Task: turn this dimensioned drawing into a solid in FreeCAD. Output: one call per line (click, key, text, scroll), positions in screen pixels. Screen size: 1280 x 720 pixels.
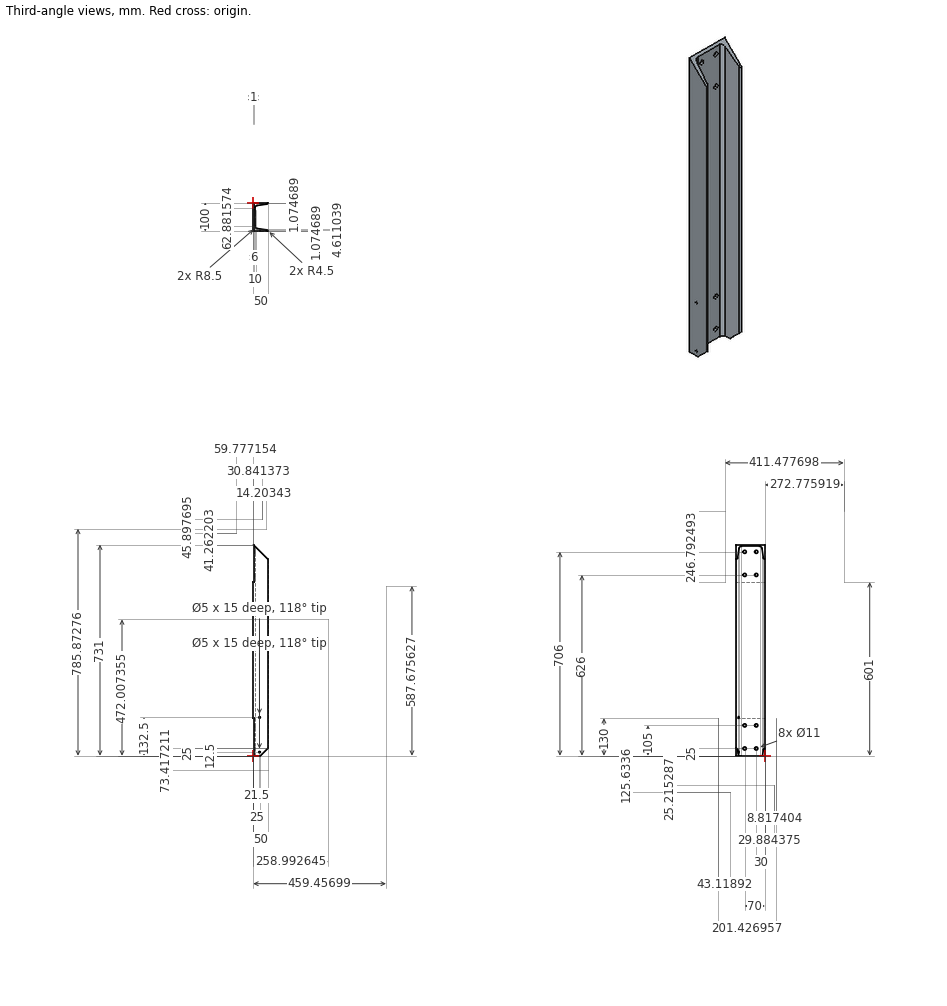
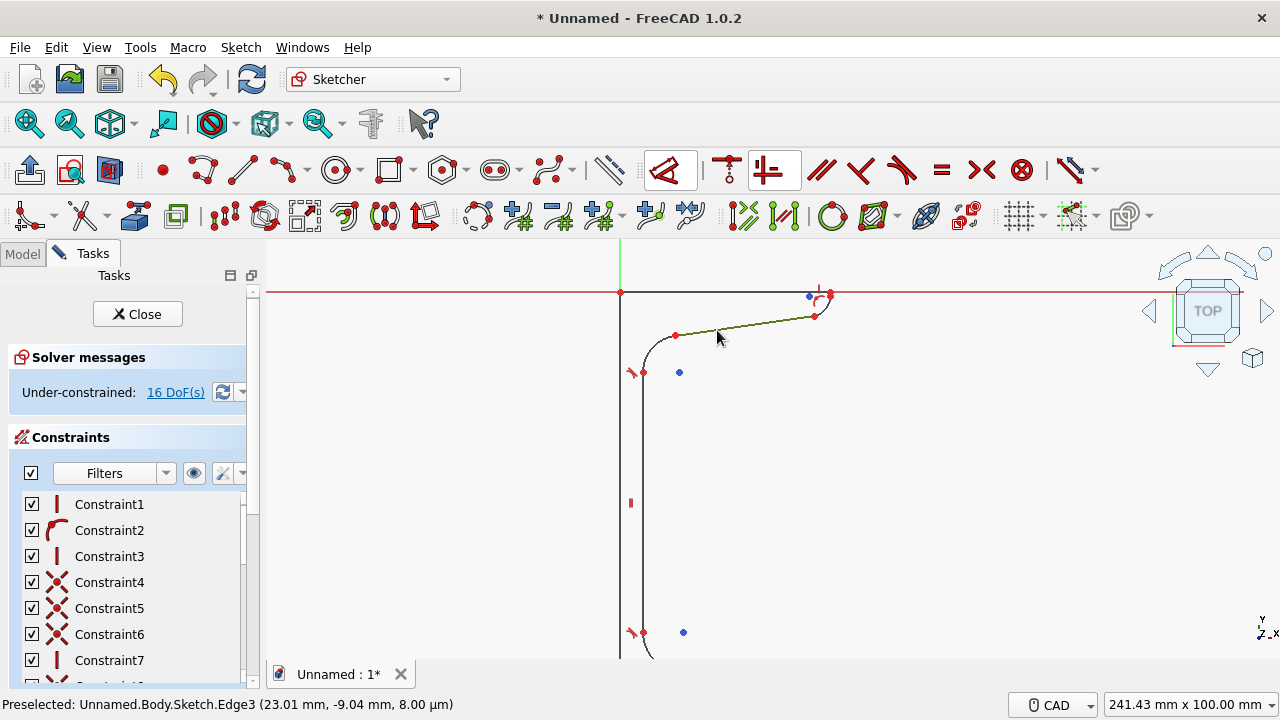
click(660, 341)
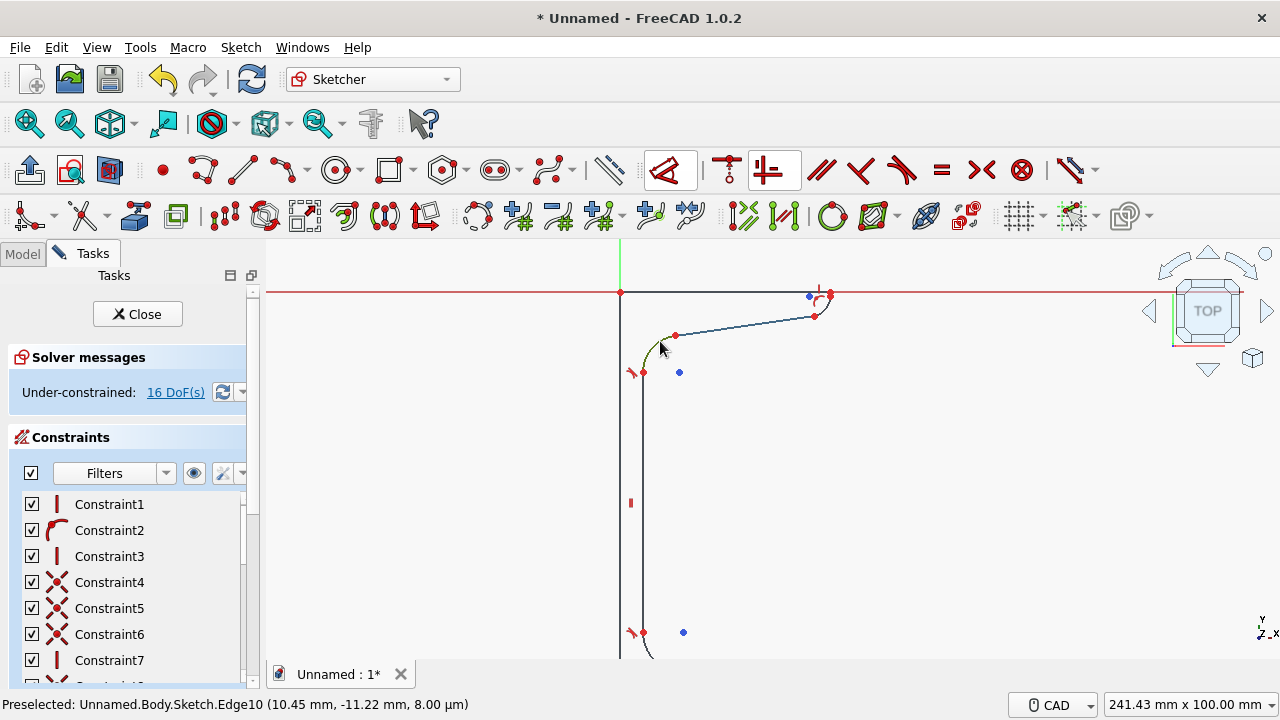
key(t)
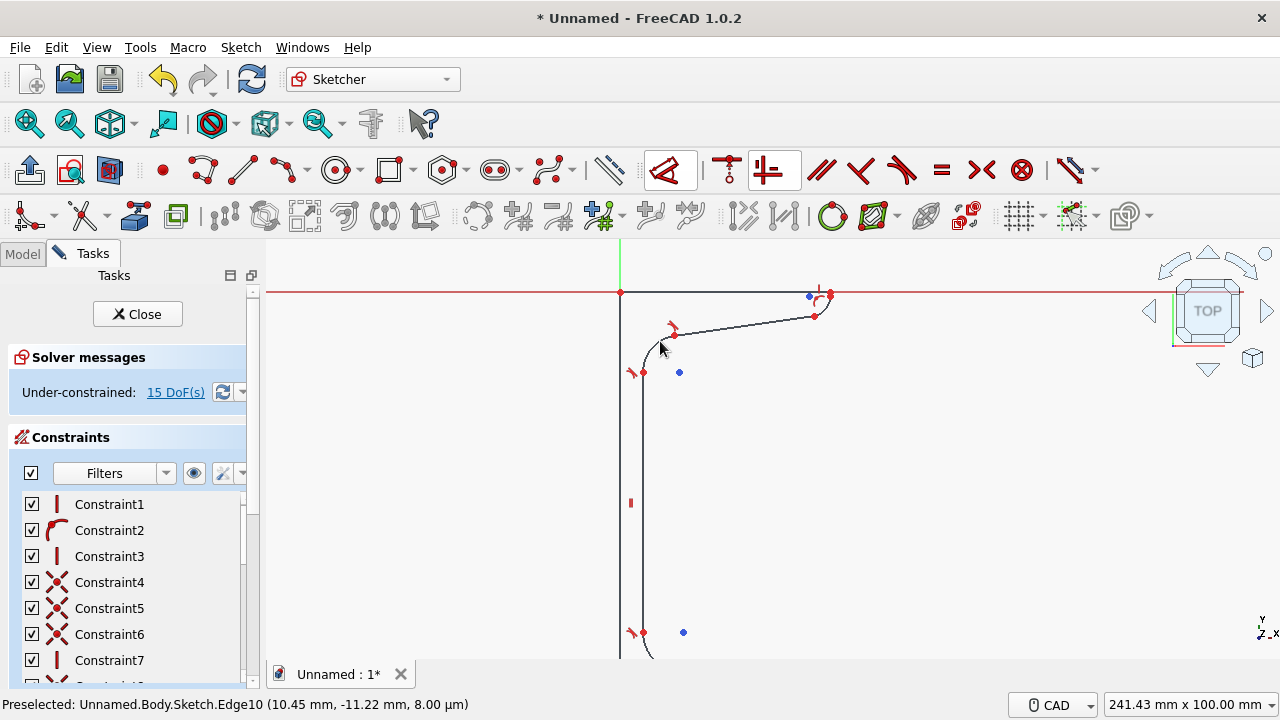
click(716, 330)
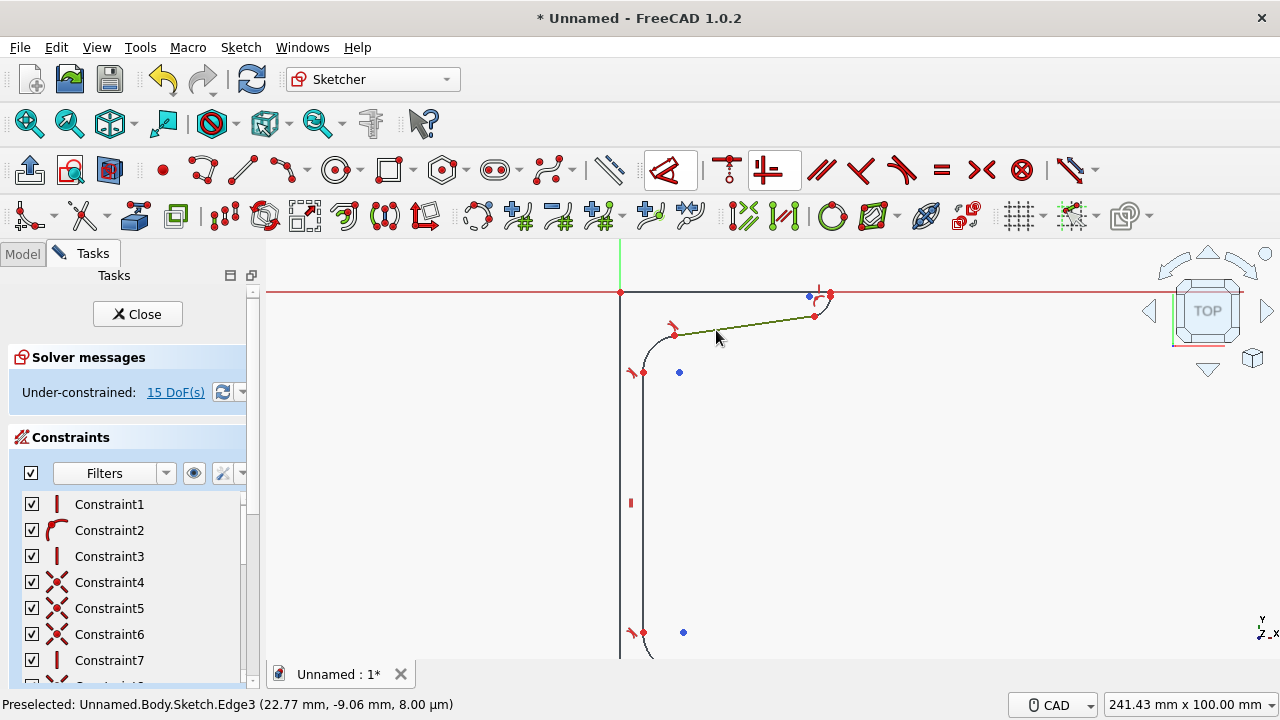
click(825, 309)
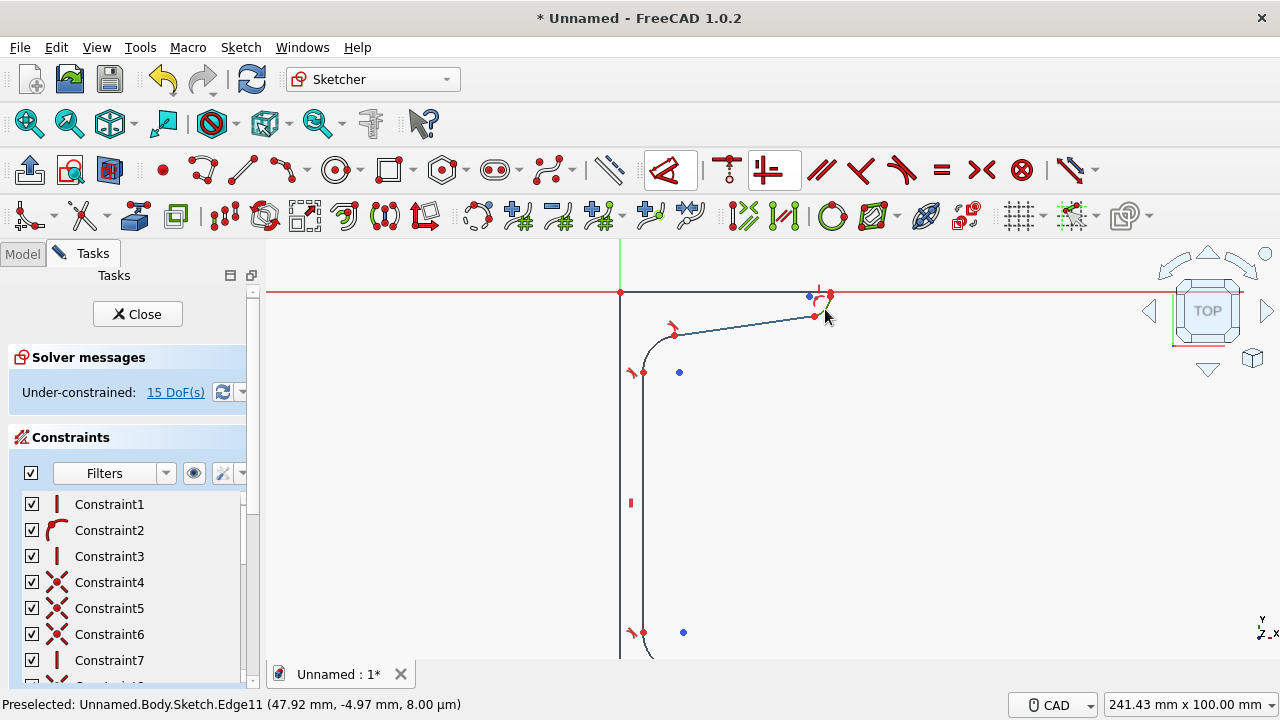
key(t)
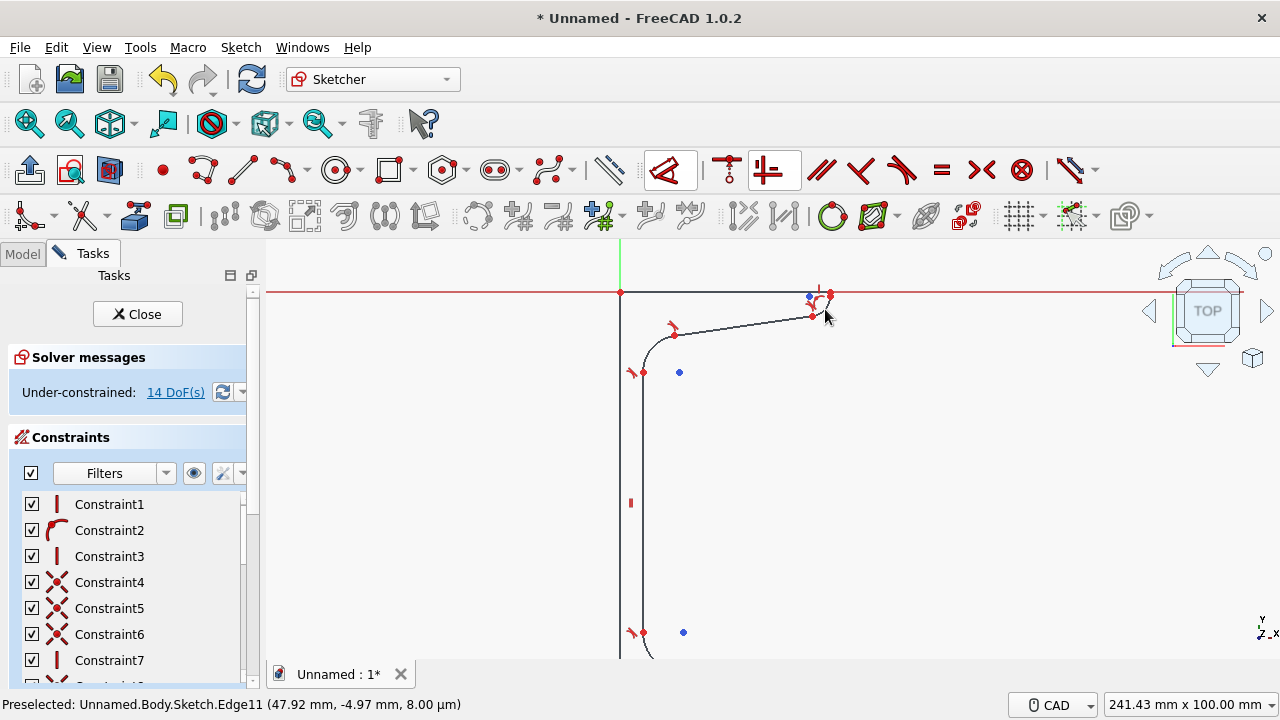
scroll(830, 294, up, 9)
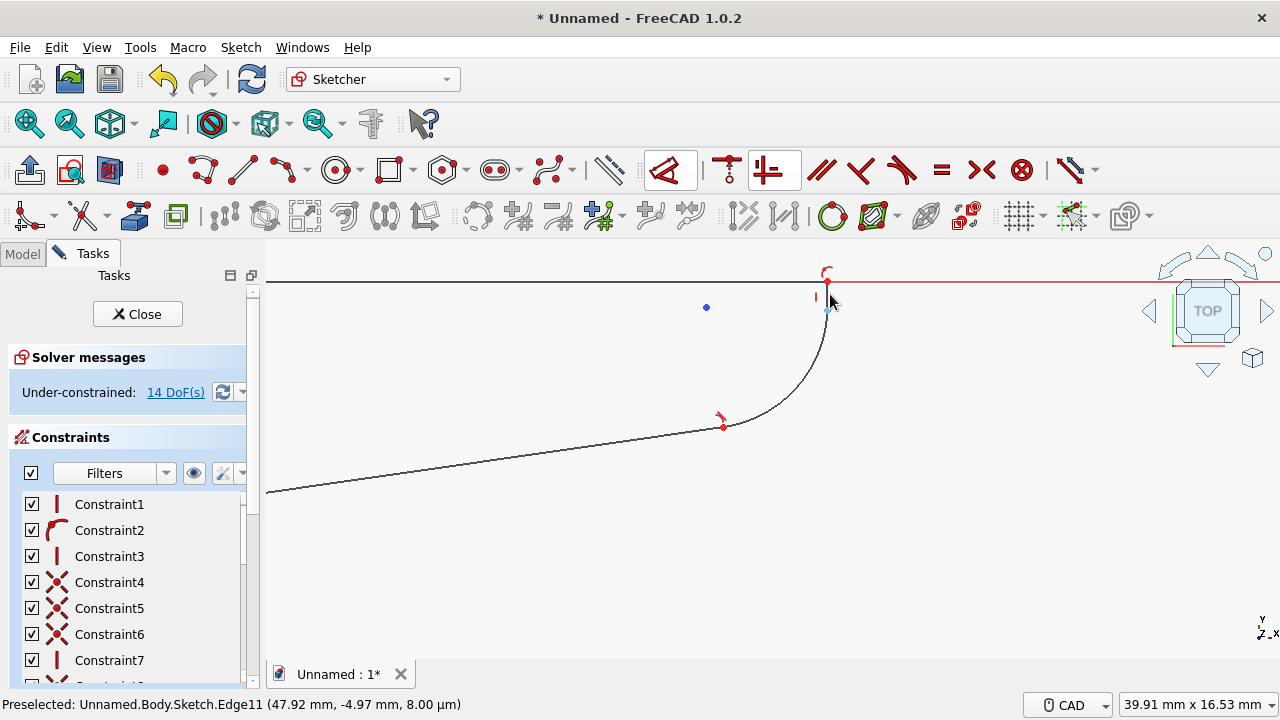
click(827, 296)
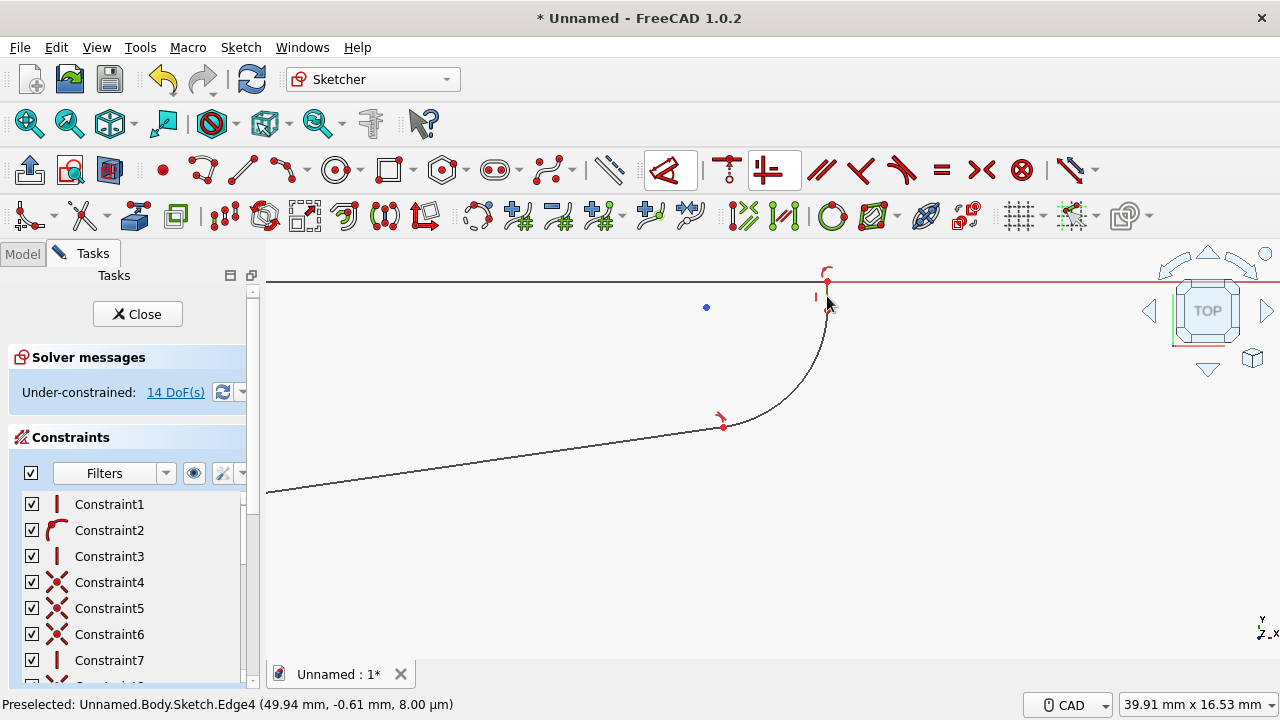
scroll(768, 312, down, 11)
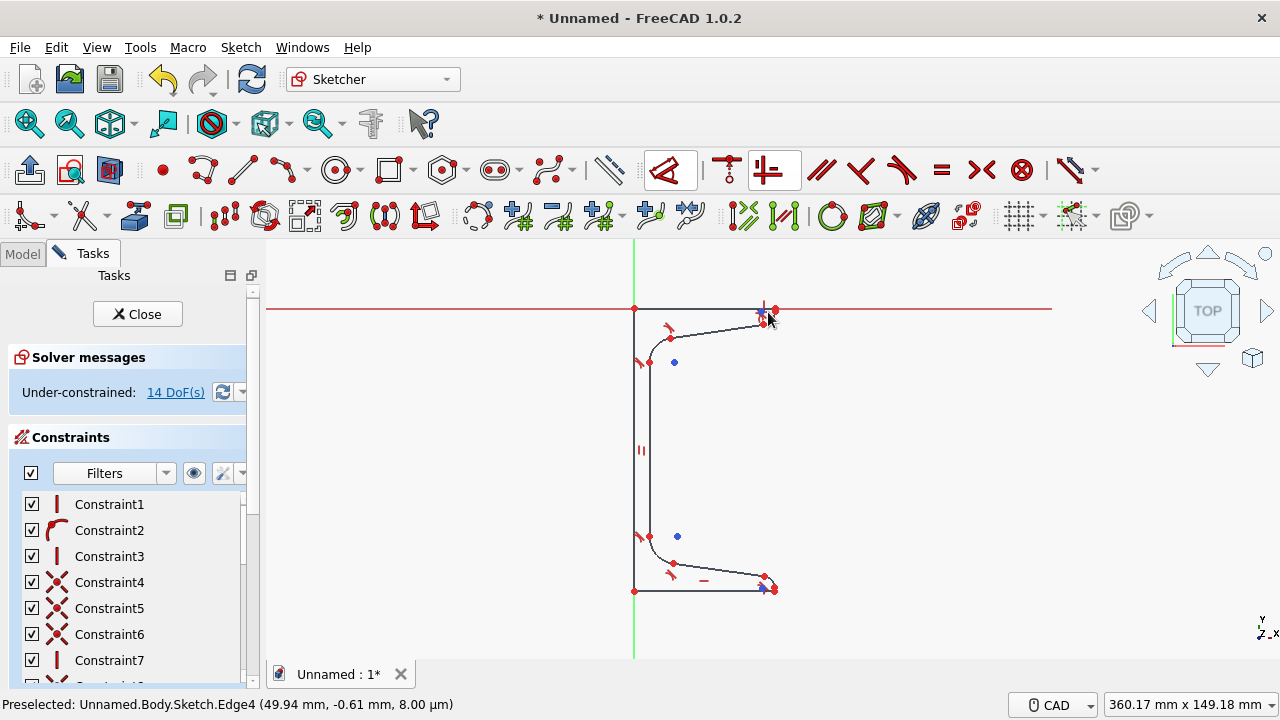
scroll(769, 323, up, 5)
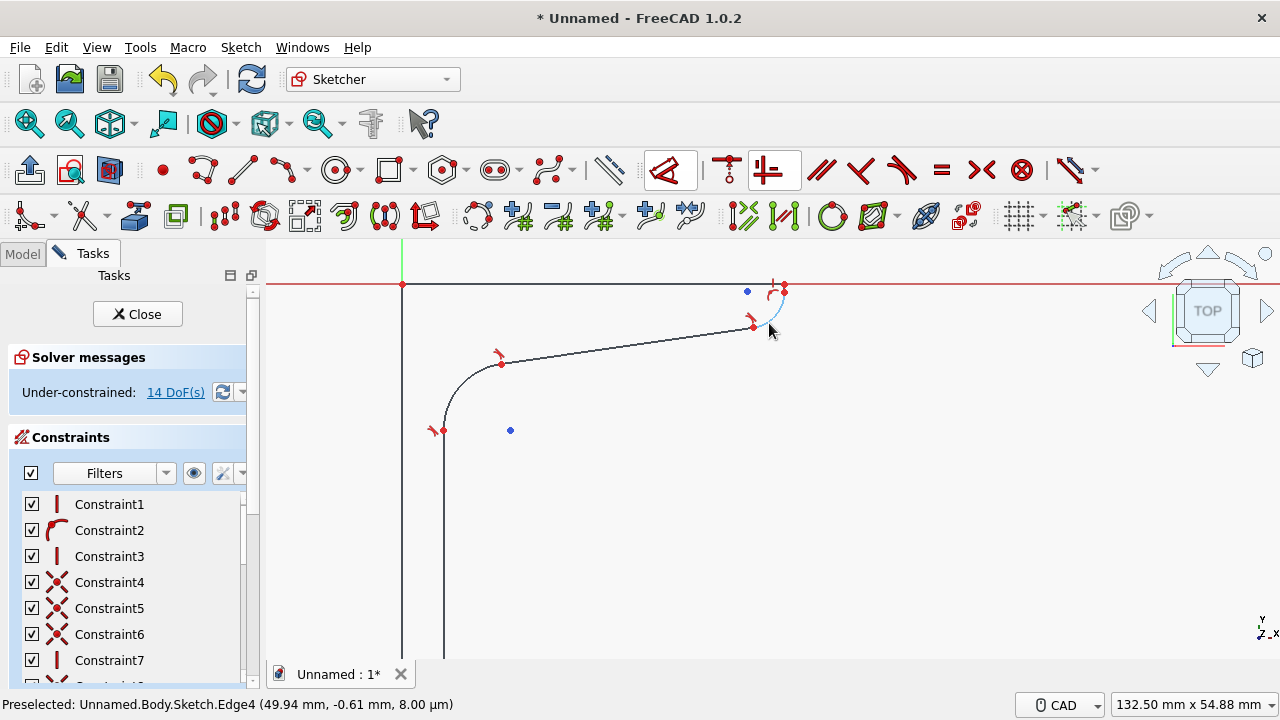
click(767, 323)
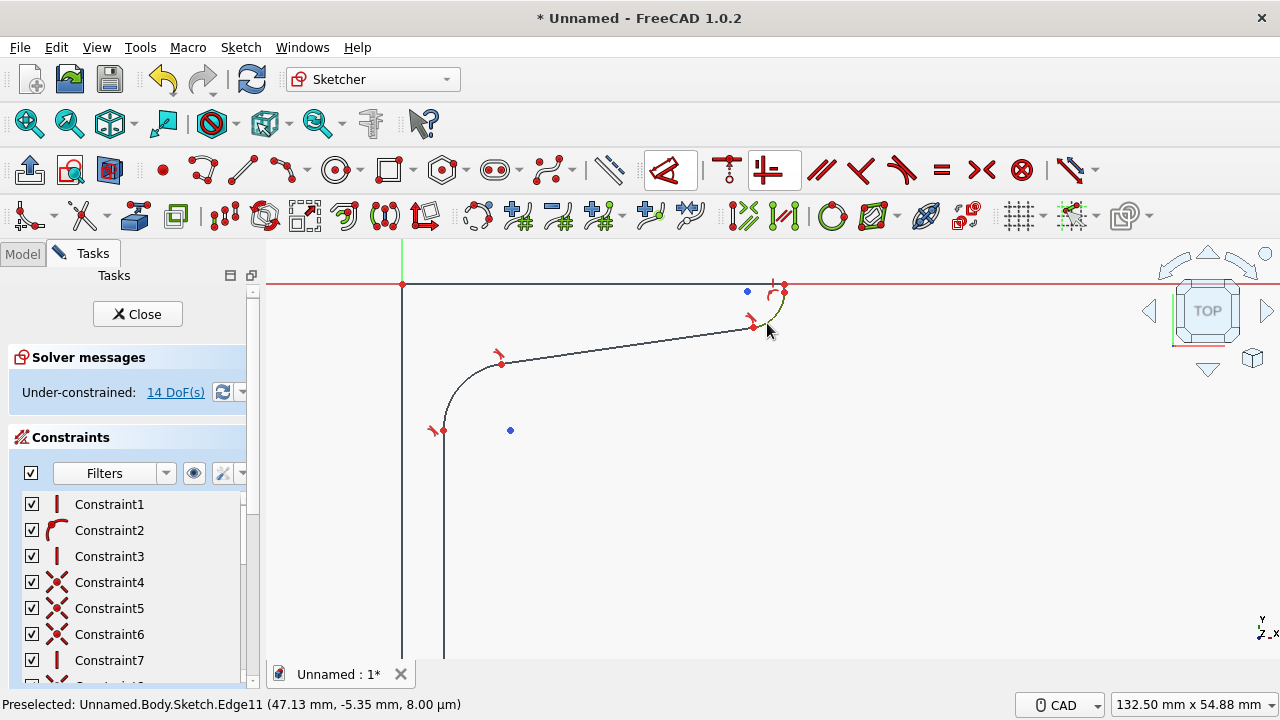
key(t)